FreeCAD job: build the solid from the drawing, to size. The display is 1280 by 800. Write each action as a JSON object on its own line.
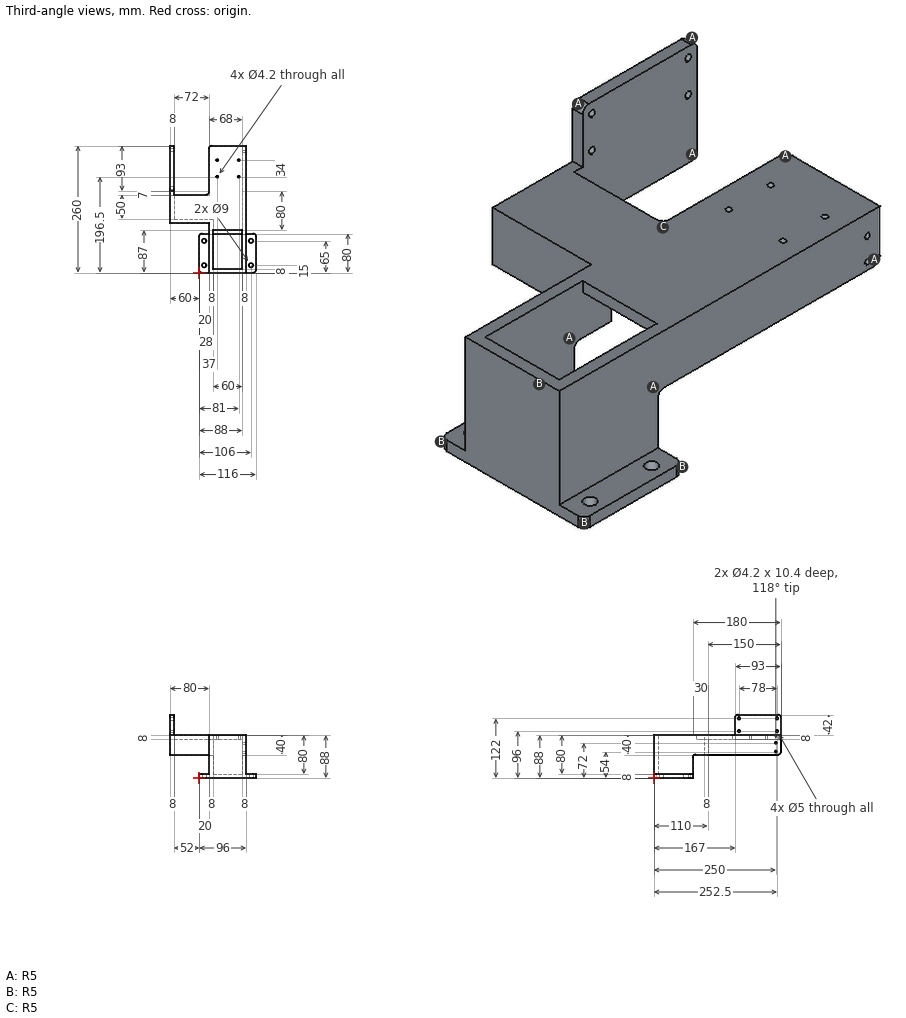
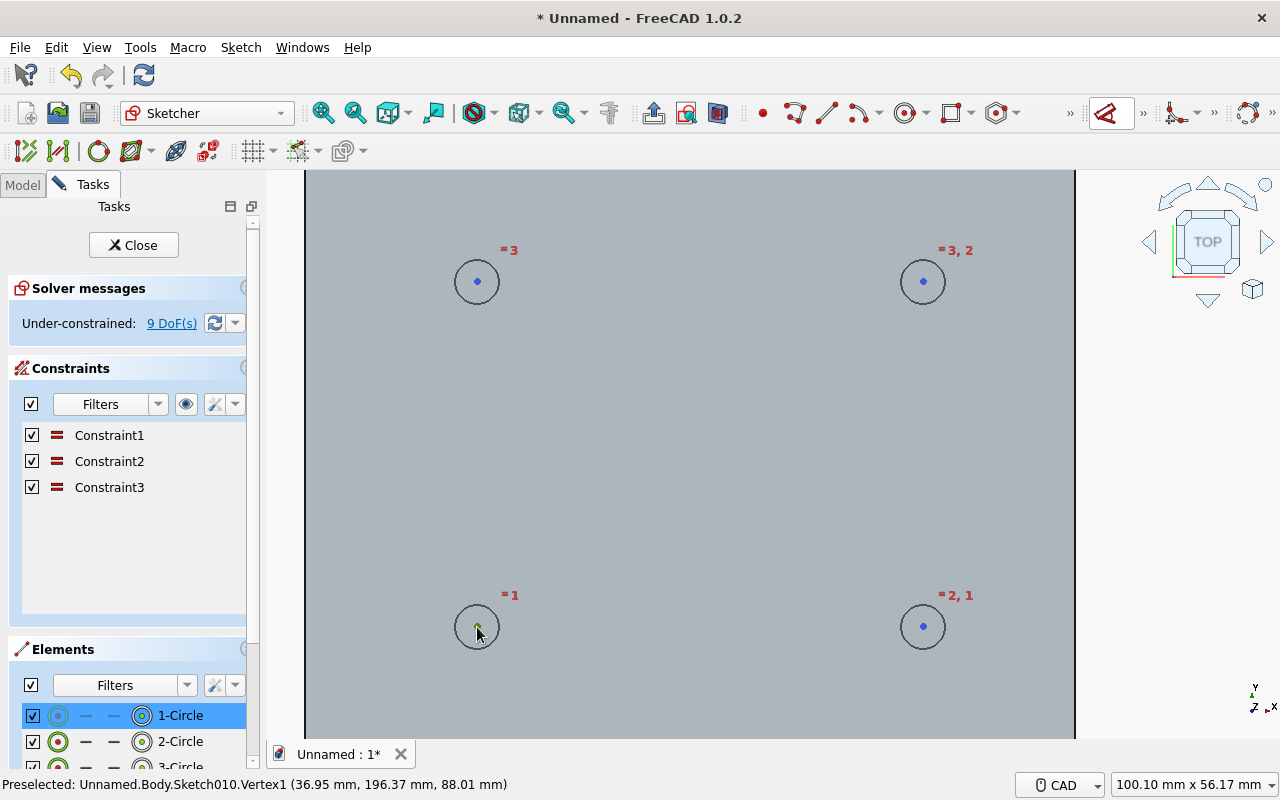
{"action": "left_click", "coordinate": [923, 627]}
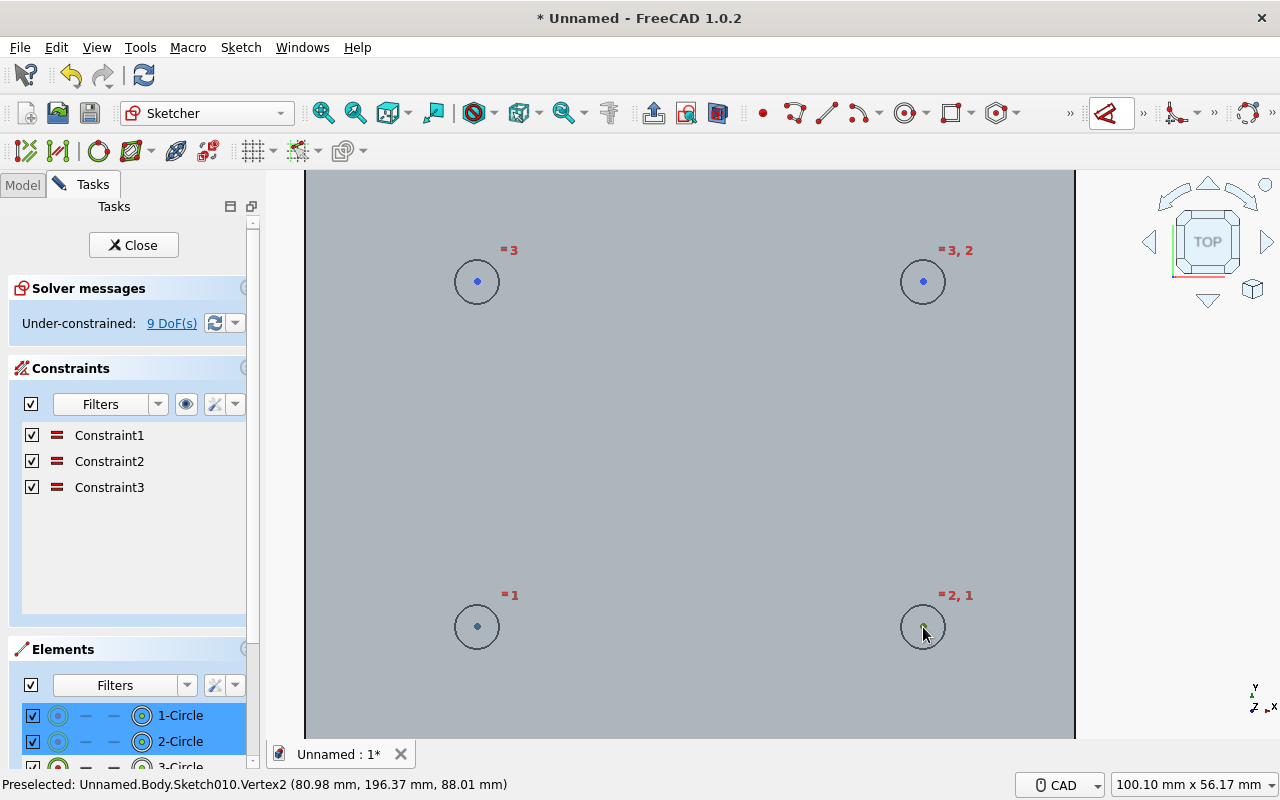
{"action": "key", "text": "h"}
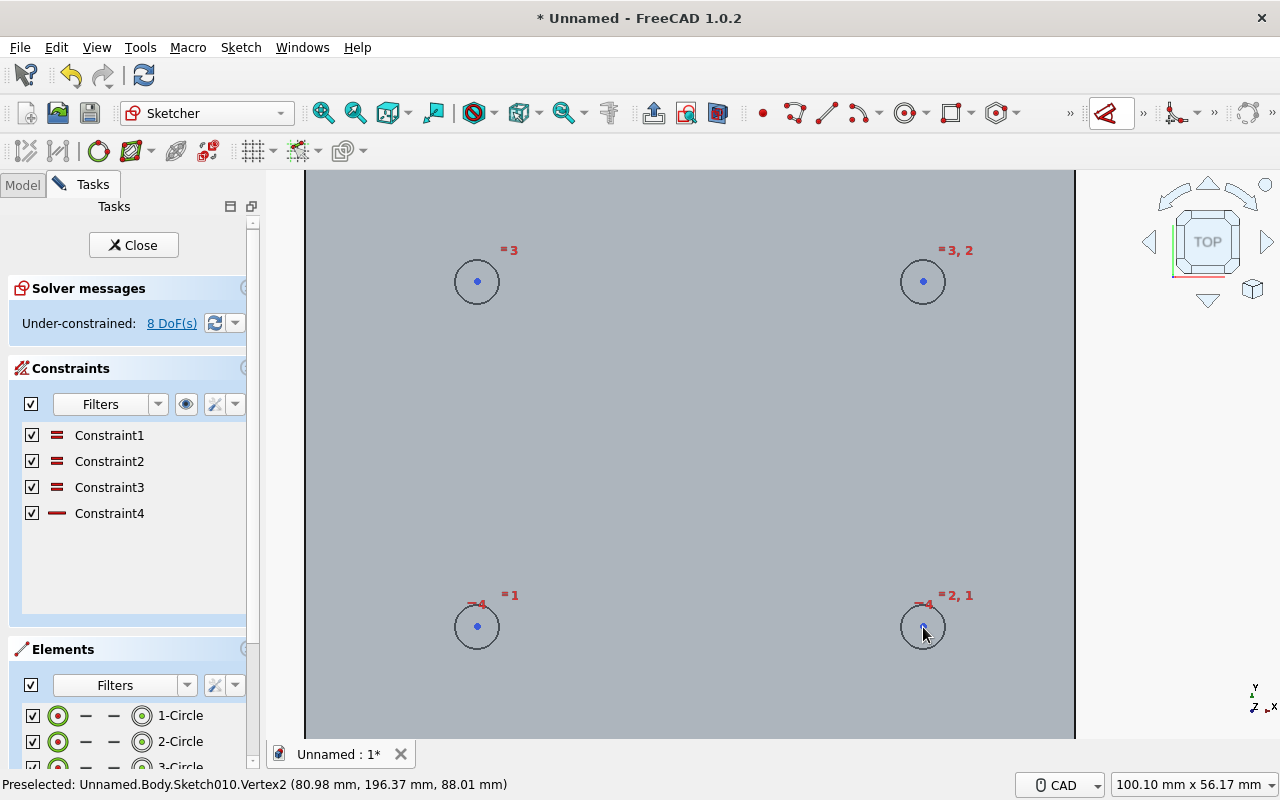
{"action": "left_click", "coordinate": [923, 627]}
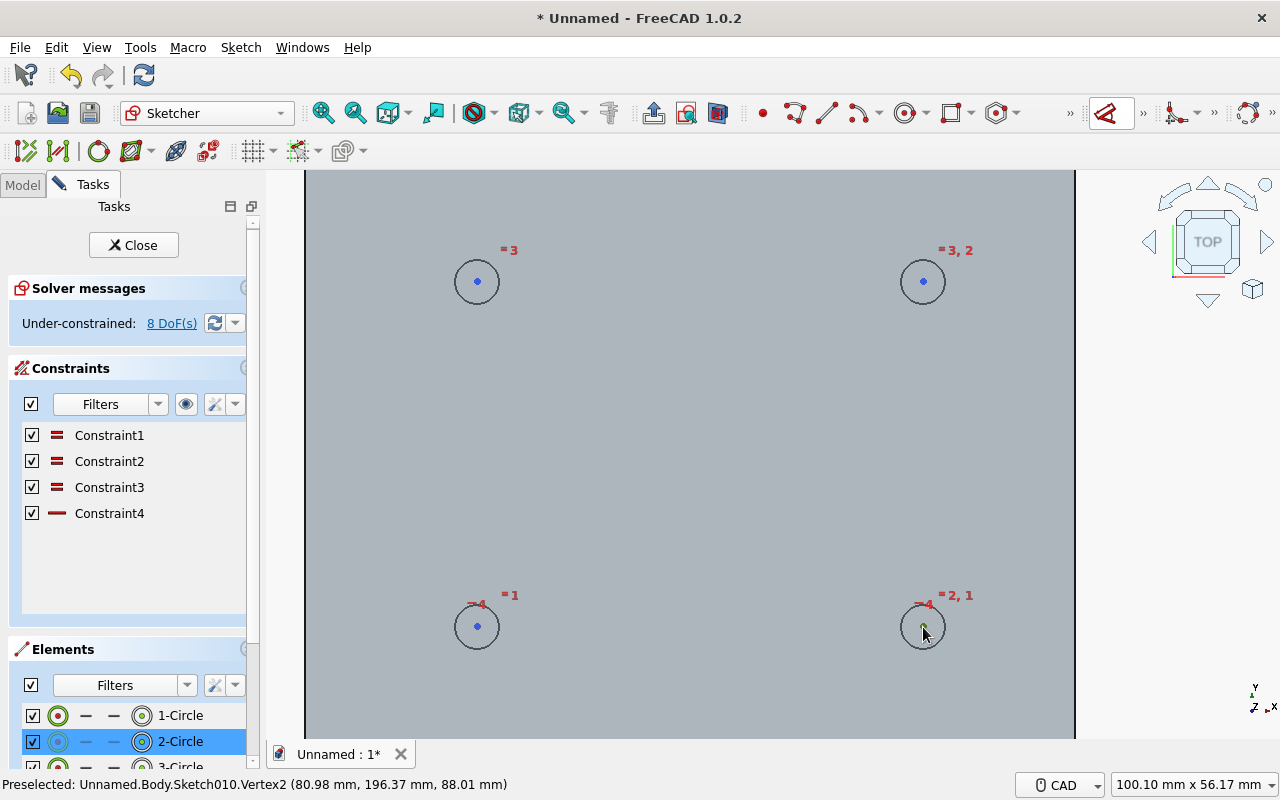
{"action": "left_click", "coordinate": [923, 282]}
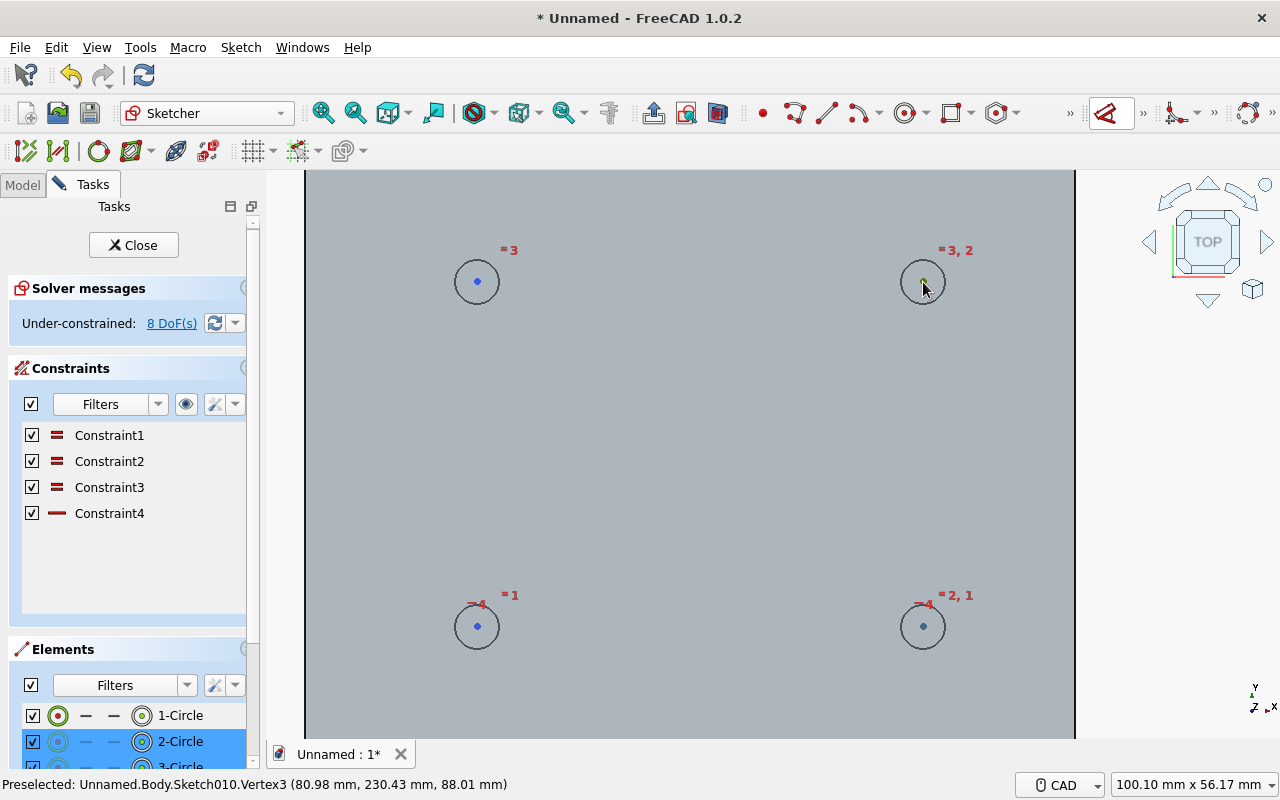
{"action": "key", "text": "v"}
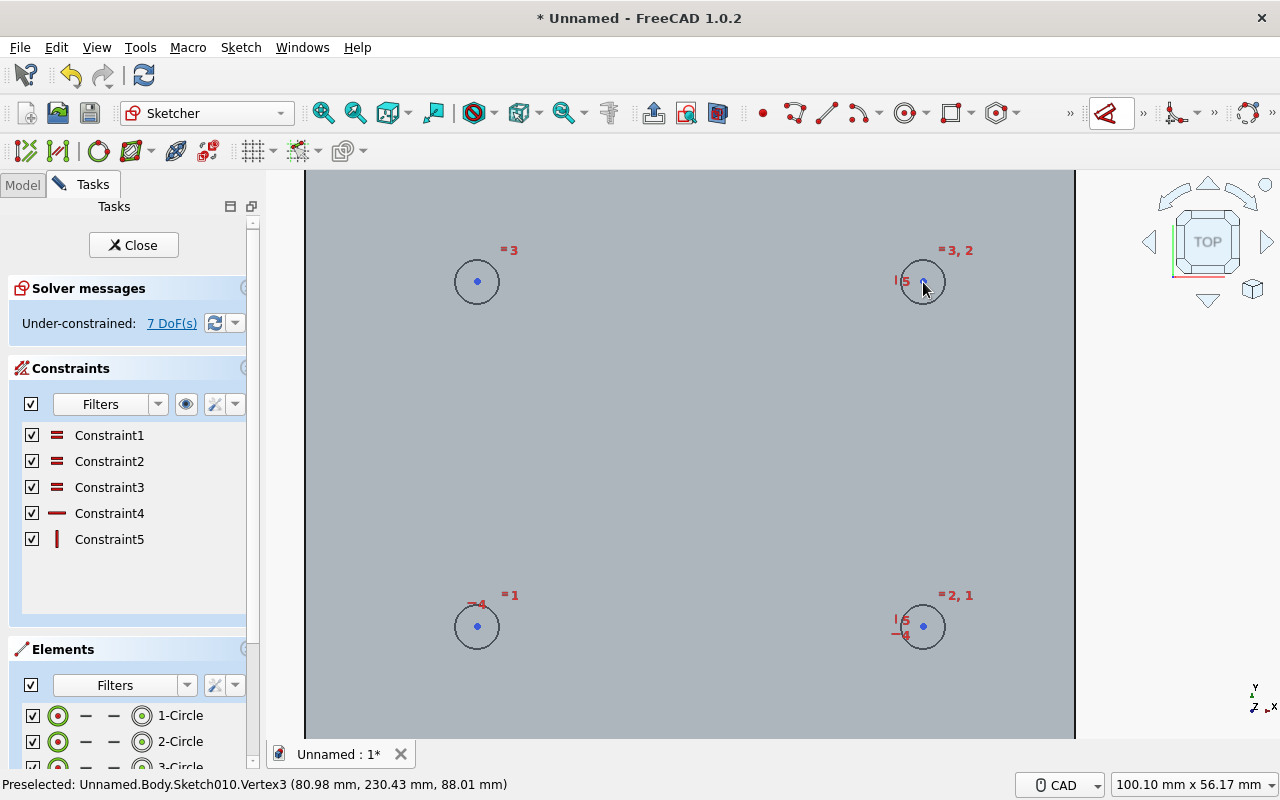
{"action": "left_click", "coordinate": [477, 627]}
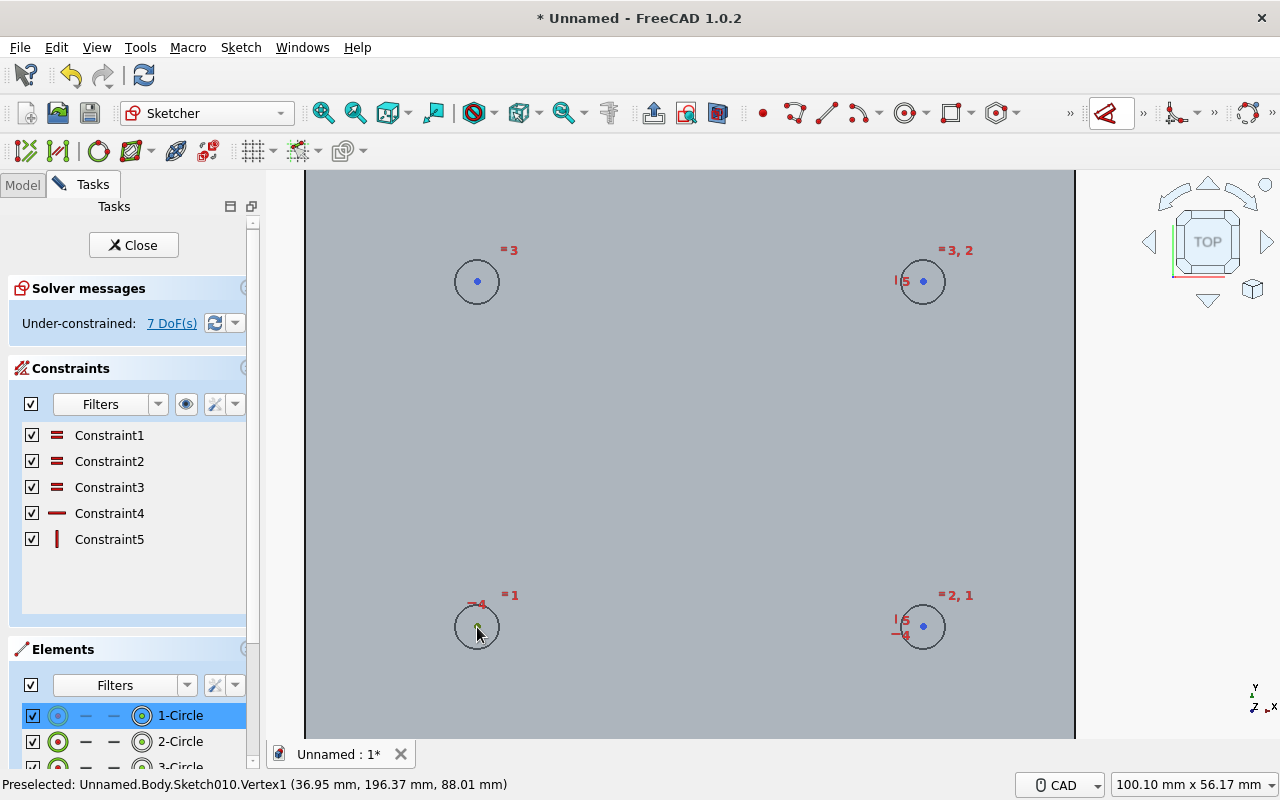
{"action": "left_click", "coordinate": [477, 282]}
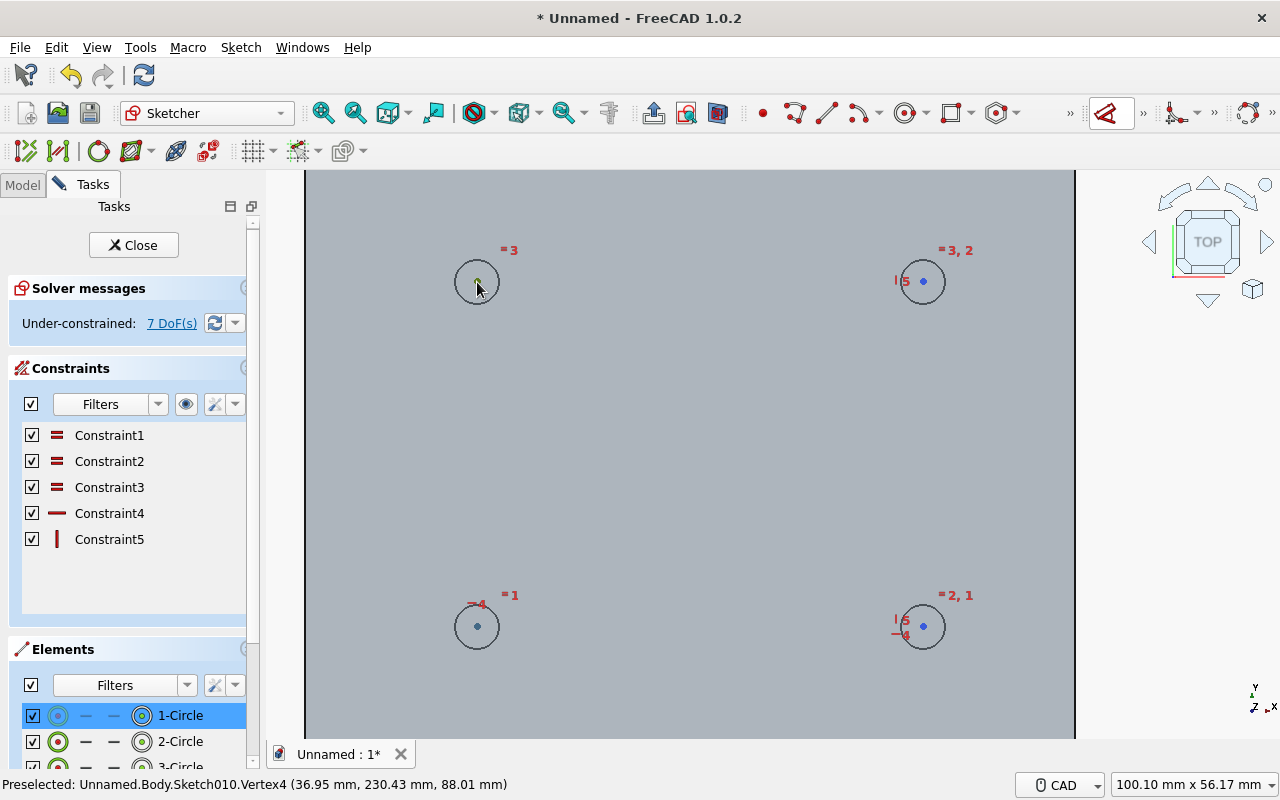
{"action": "key", "text": "v"}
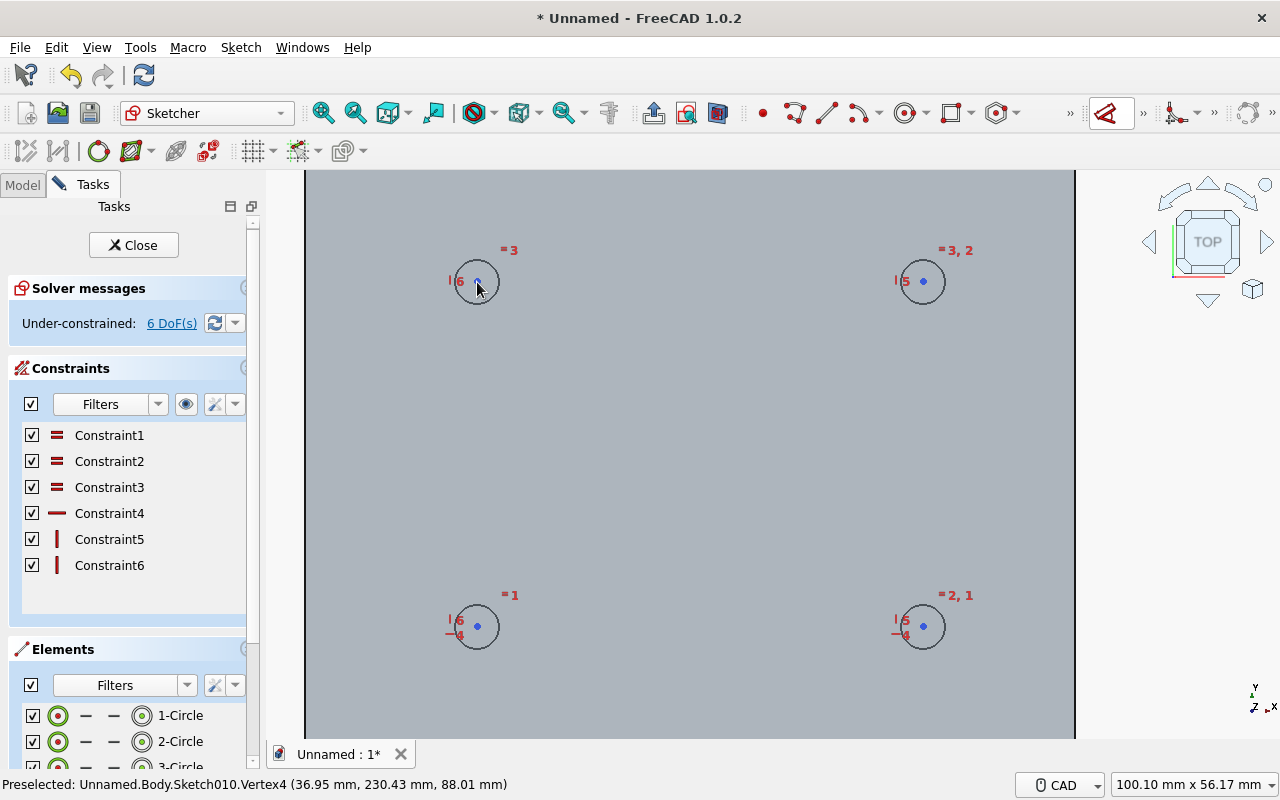
{"action": "left_click", "coordinate": [923, 282]}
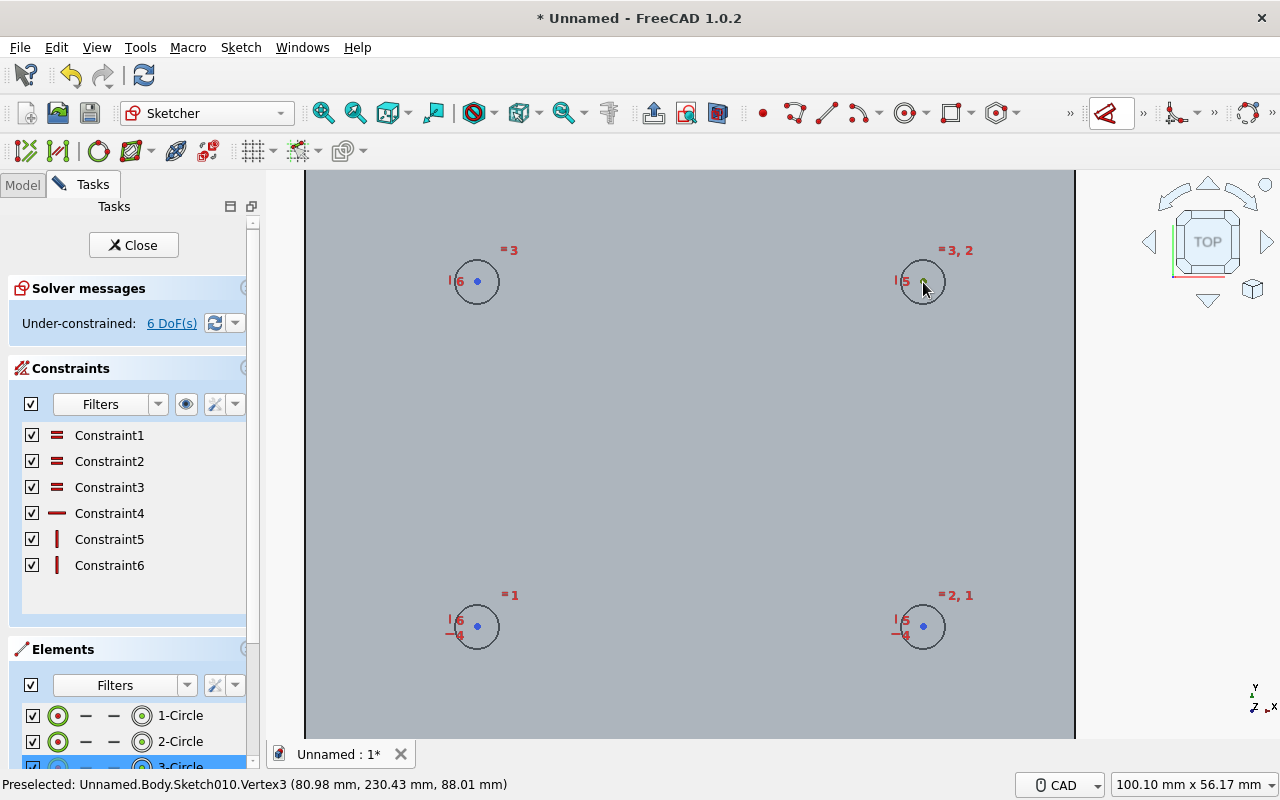
{"action": "left_click", "coordinate": [477, 282]}